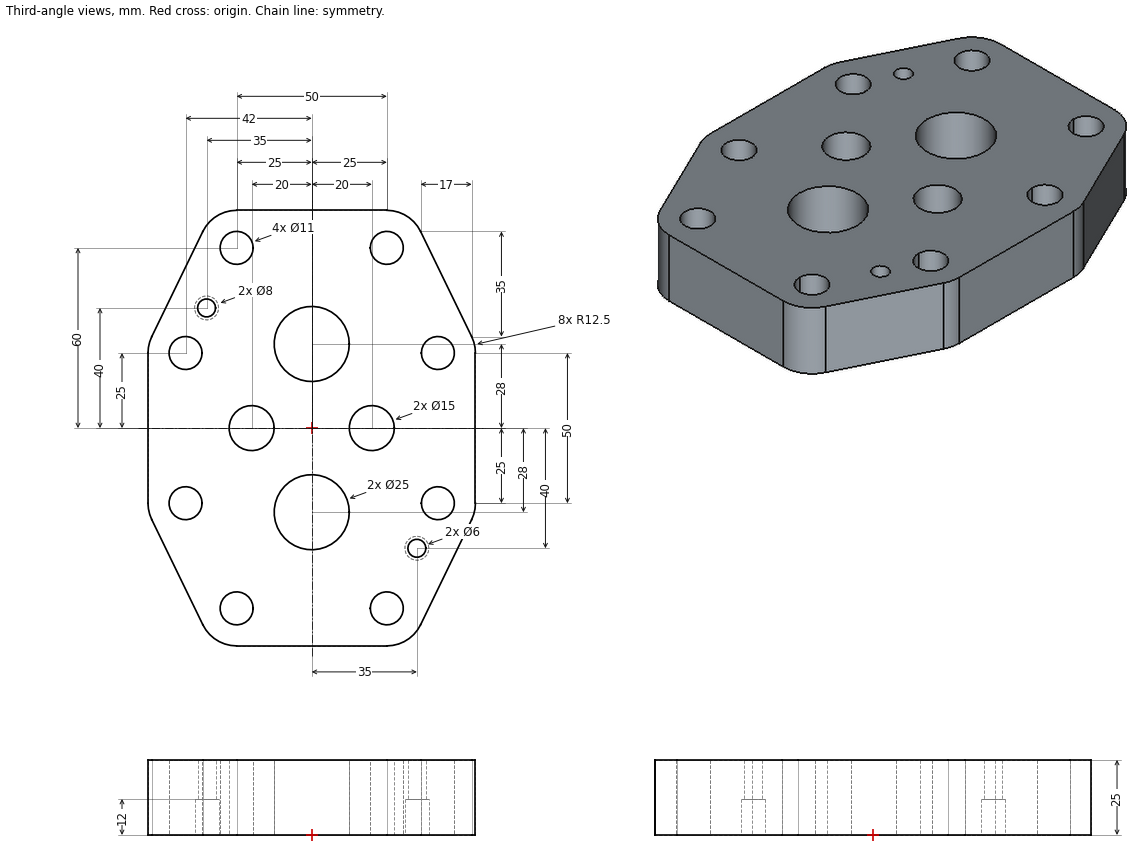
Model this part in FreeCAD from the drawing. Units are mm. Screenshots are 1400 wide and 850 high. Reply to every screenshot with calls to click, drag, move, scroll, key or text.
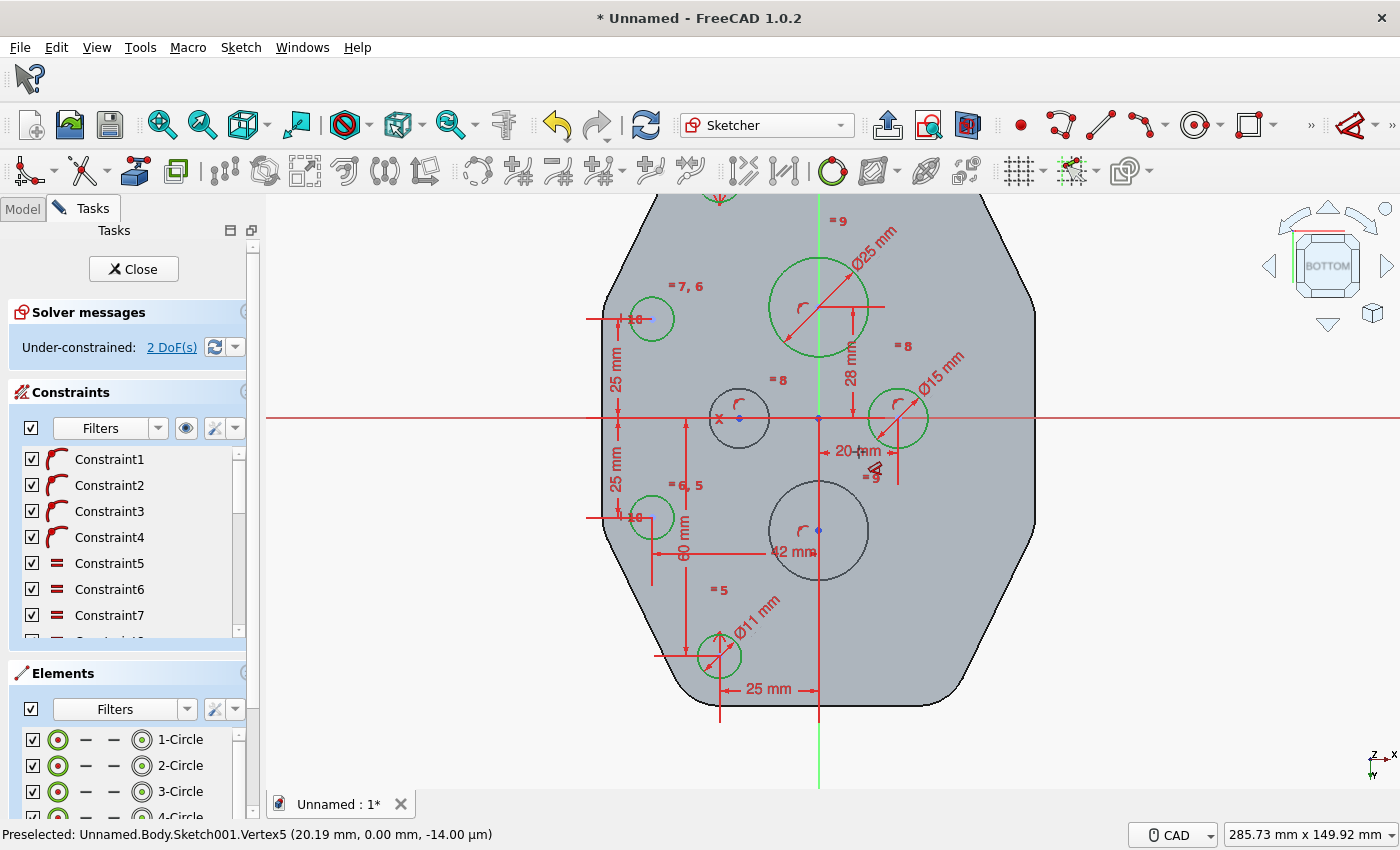
click(739, 418)
click(779, 452)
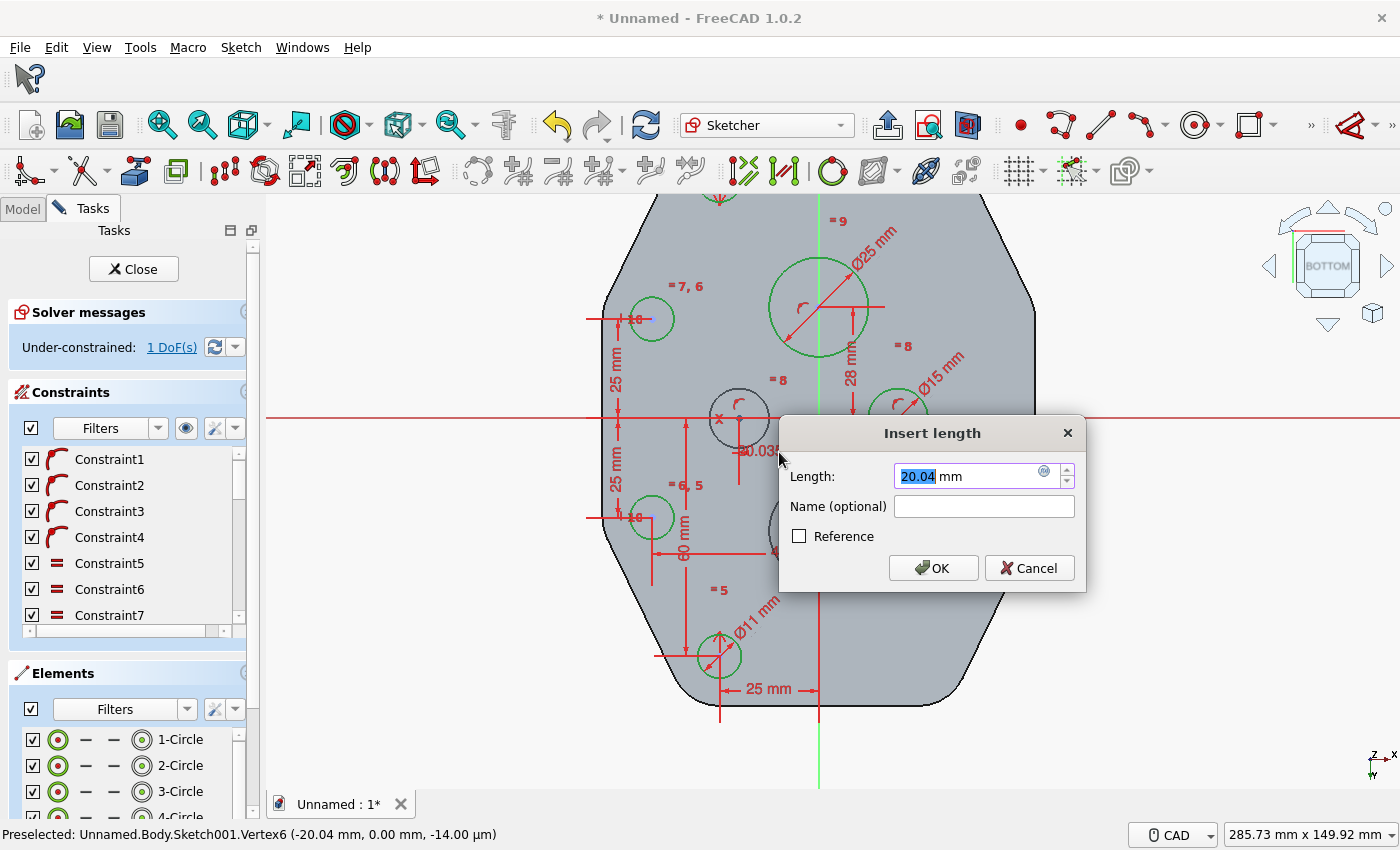
text(20)
key(Return)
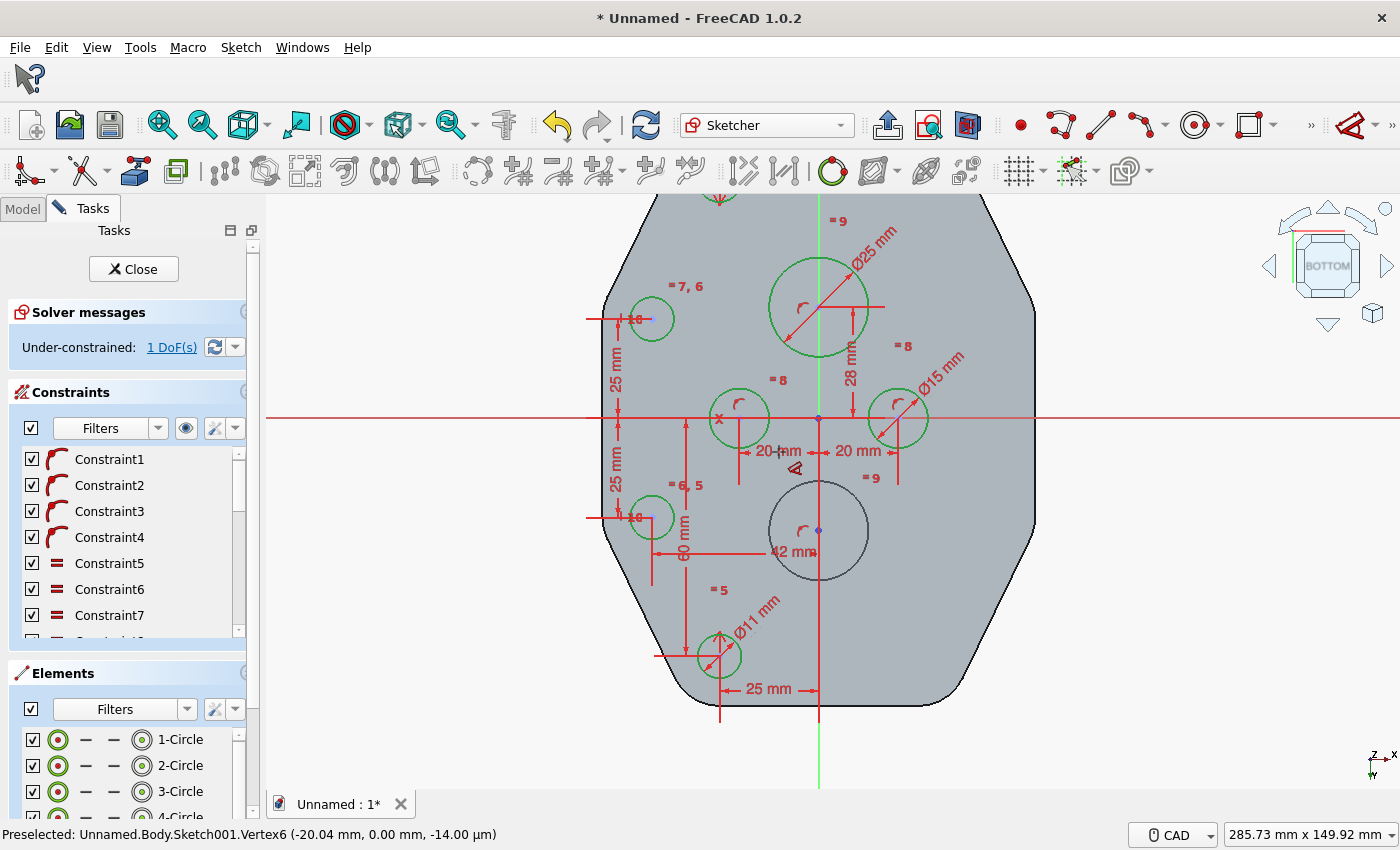
click(819, 531)
click(853, 475)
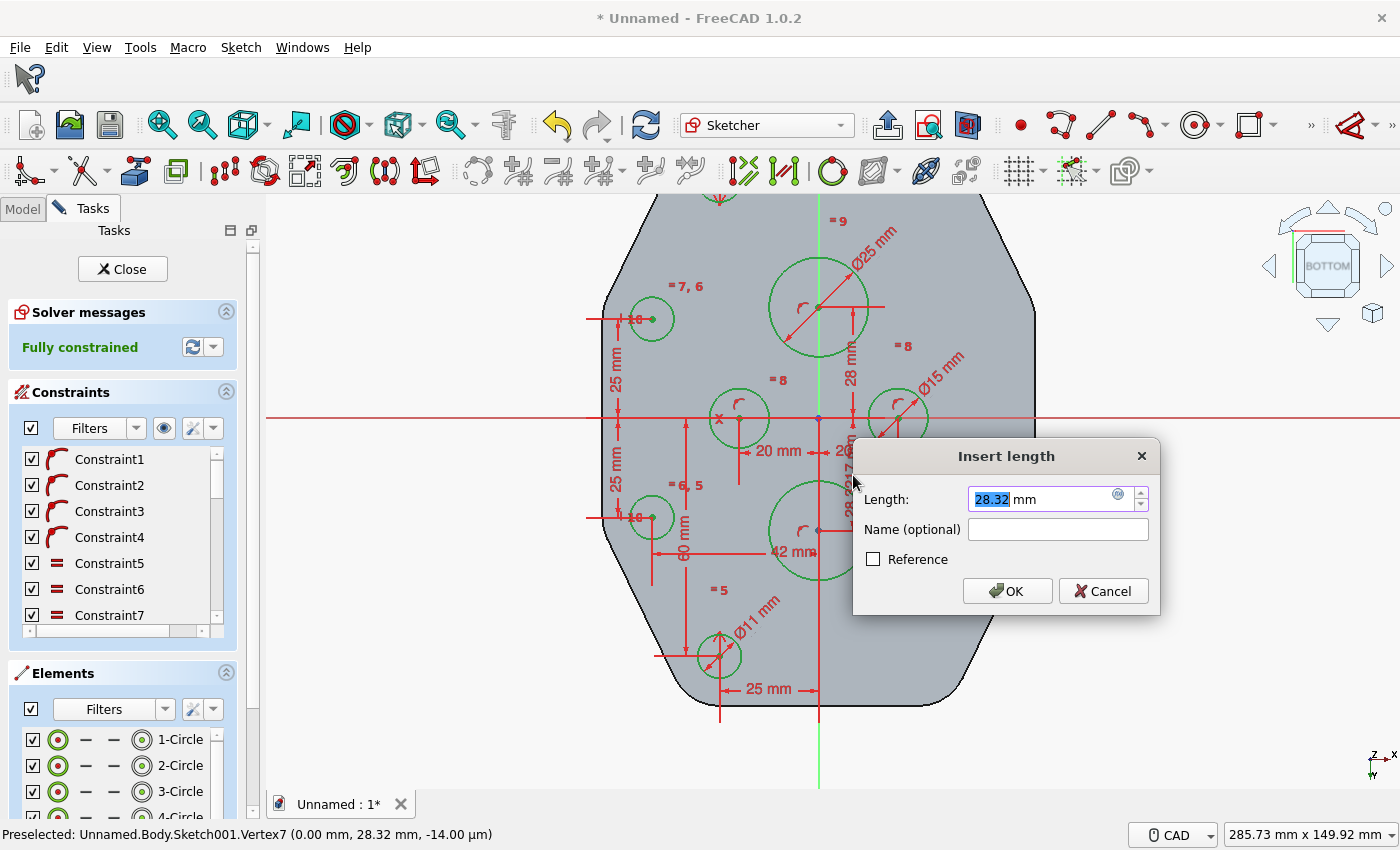
text(28)
key(Return)
key(Escape)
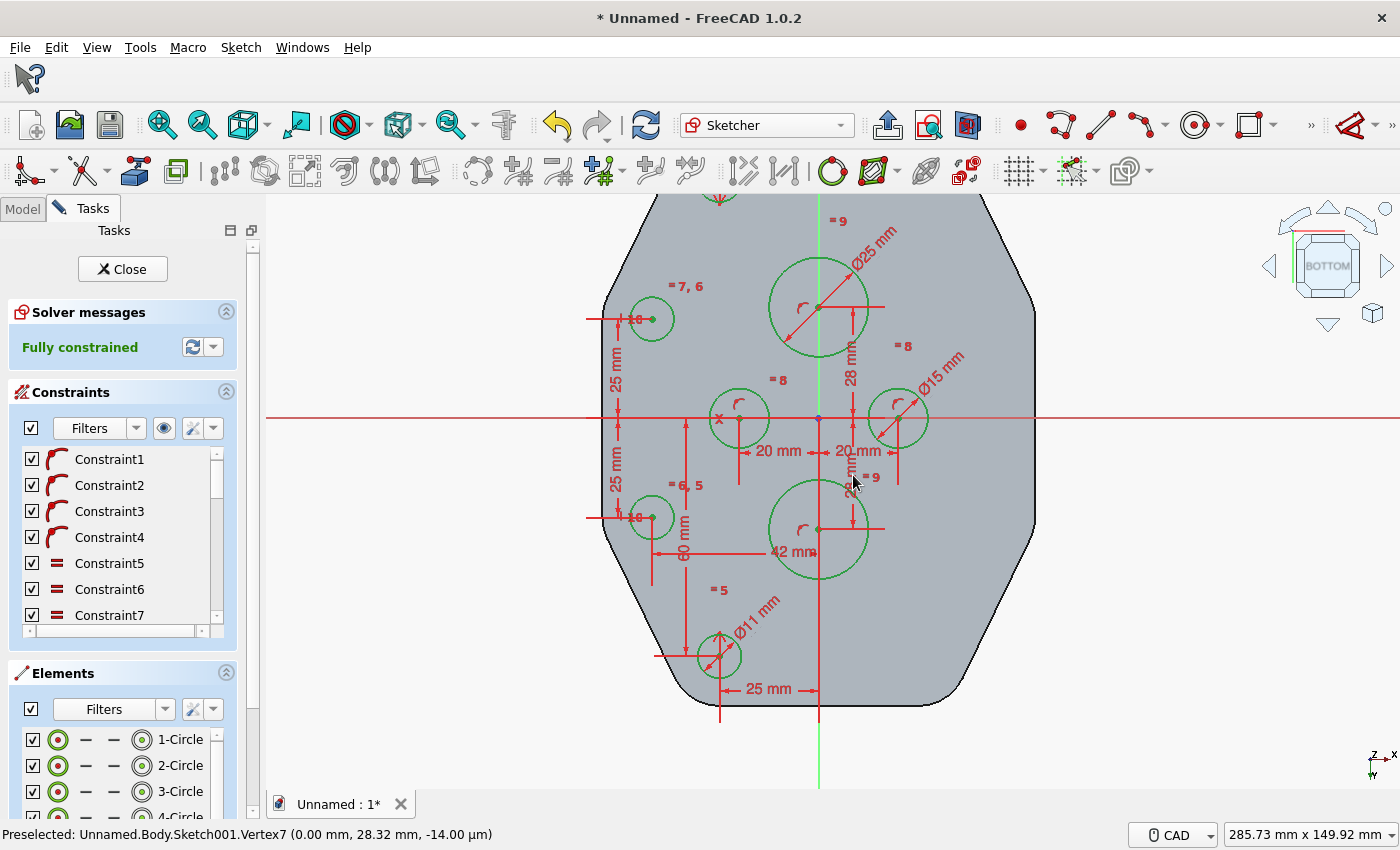
click(123, 269)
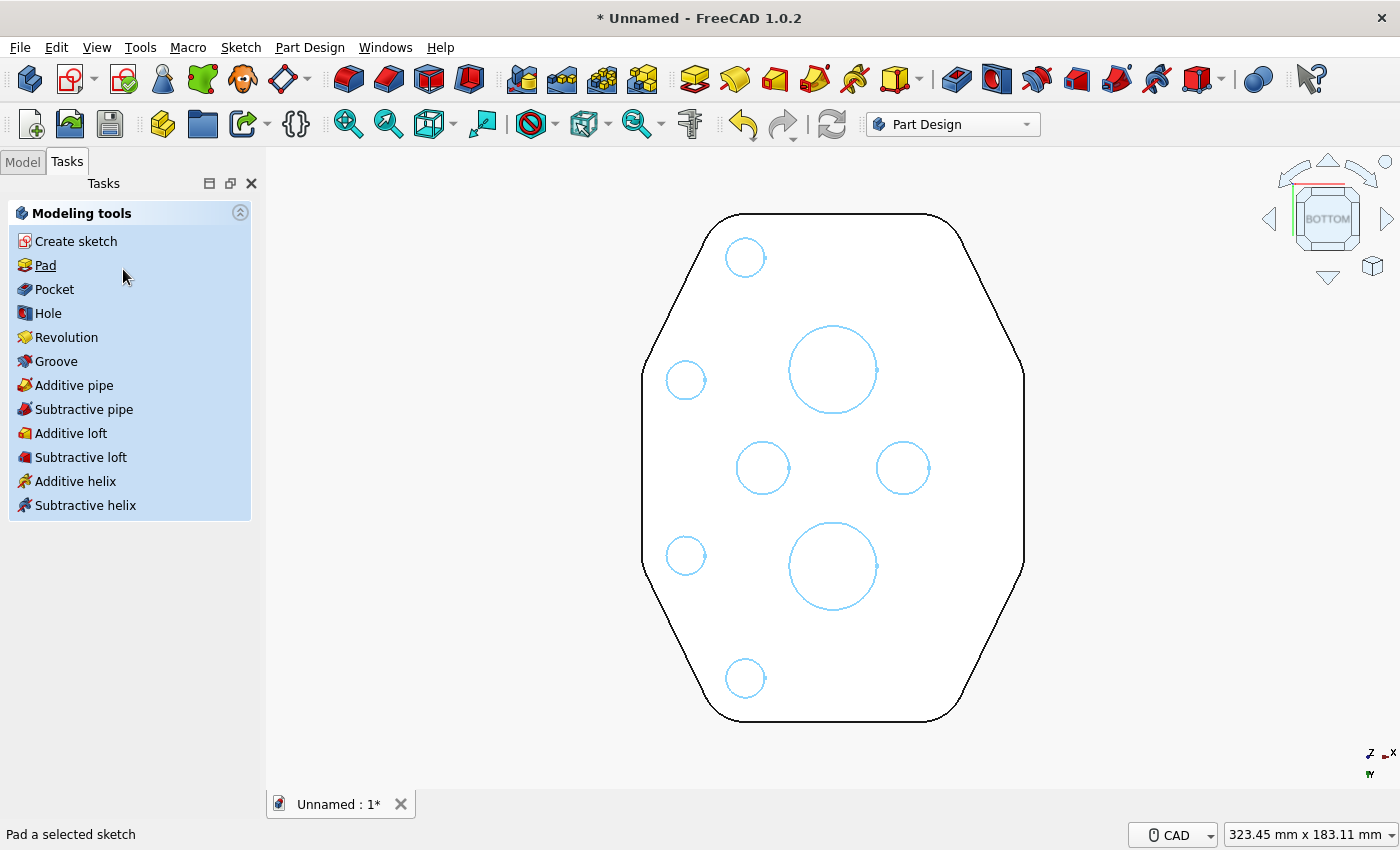
click(958, 80)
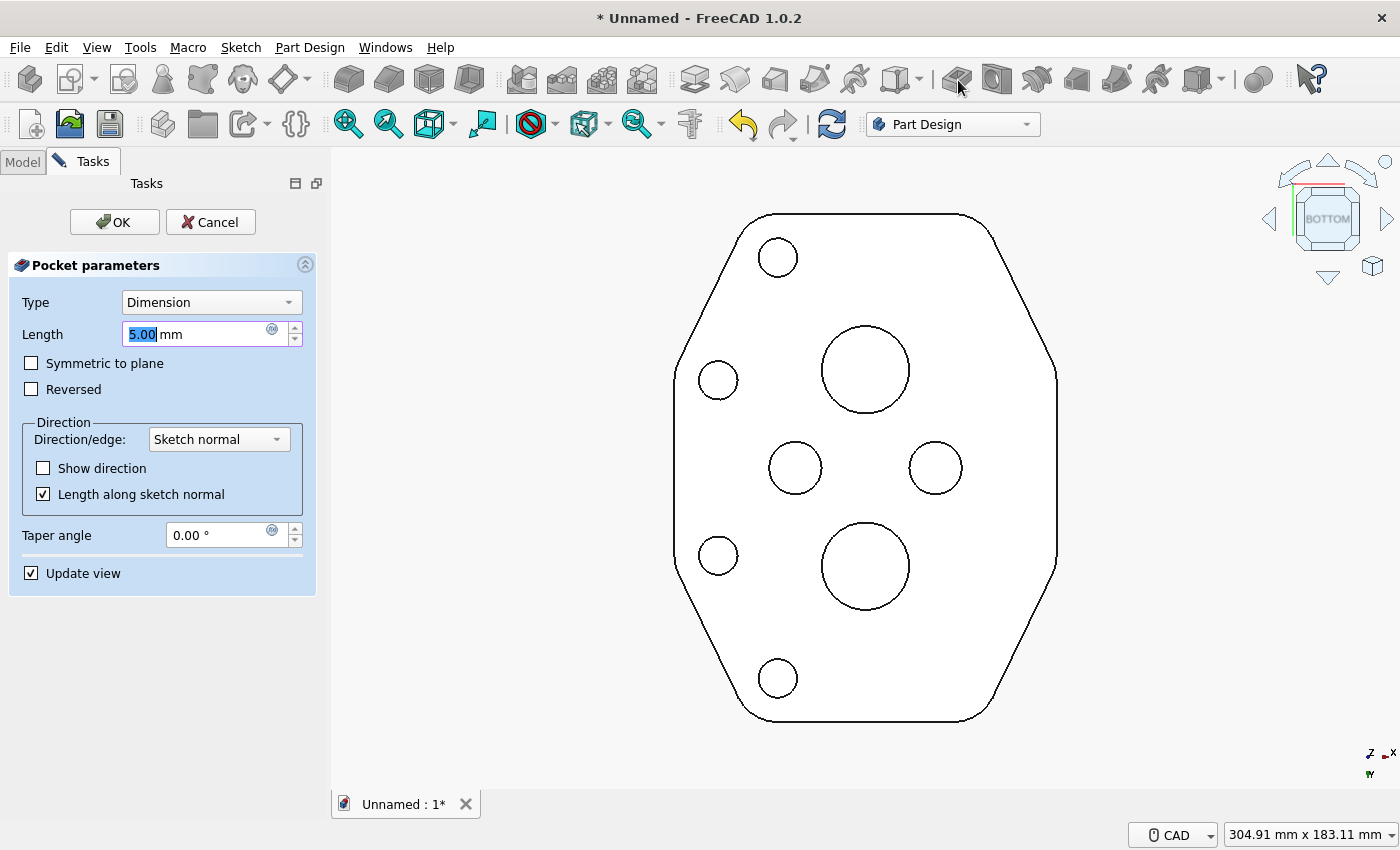
click(212, 302)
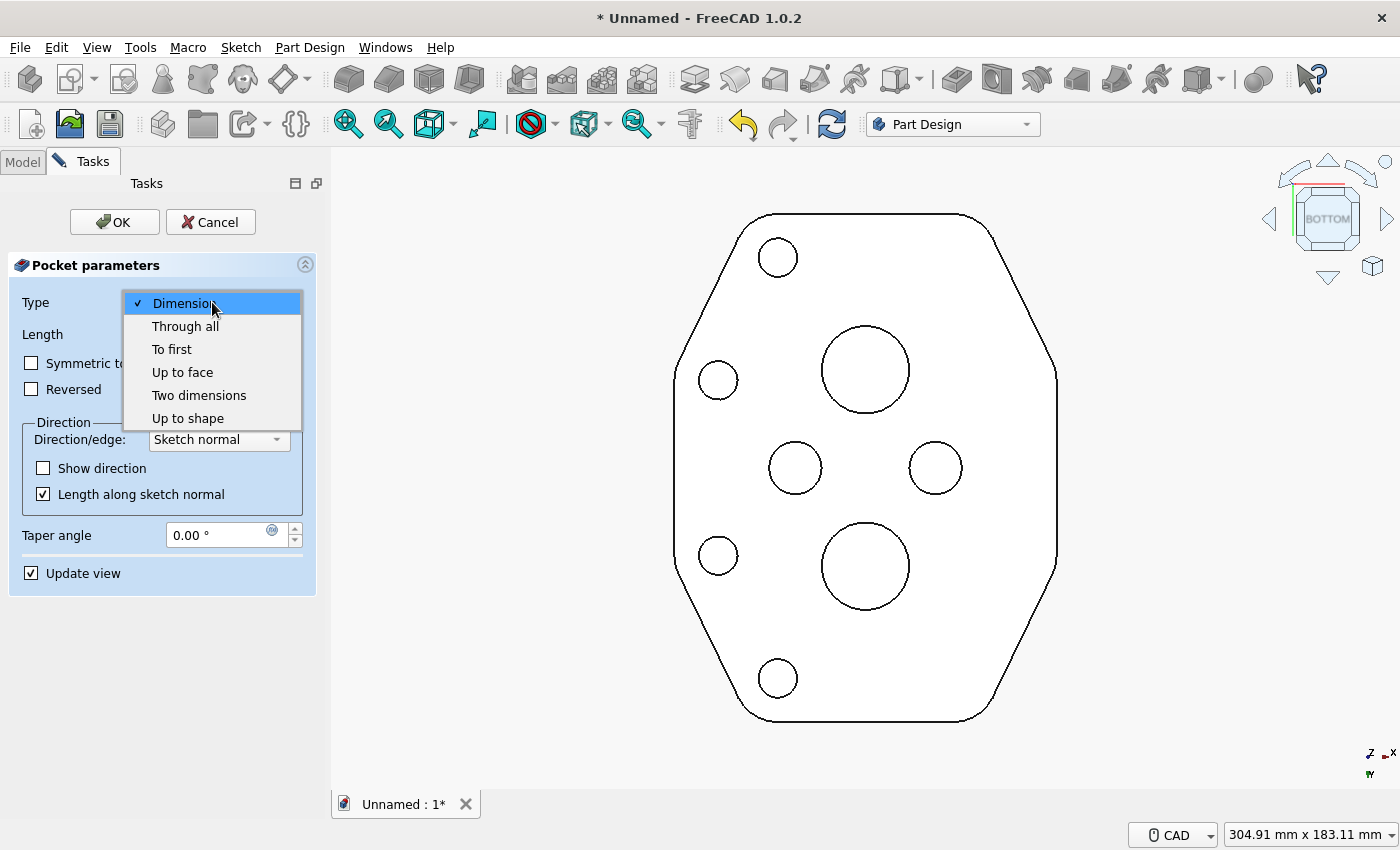
click(212, 326)